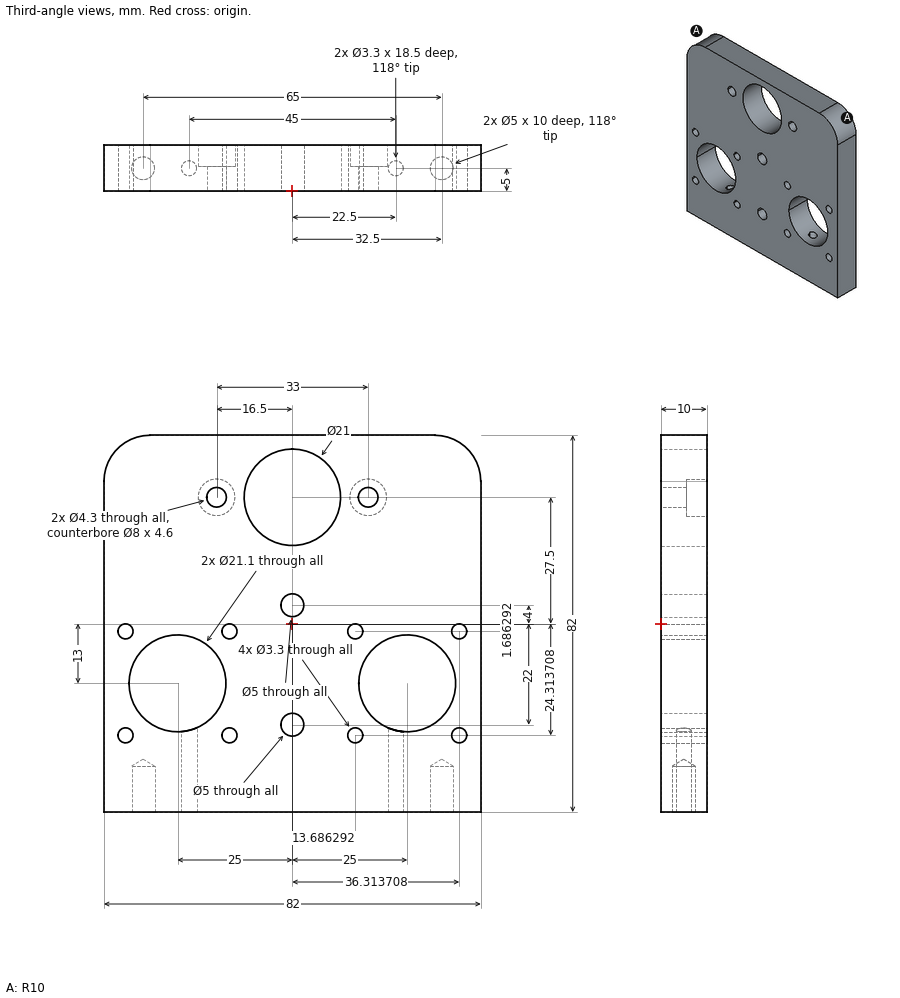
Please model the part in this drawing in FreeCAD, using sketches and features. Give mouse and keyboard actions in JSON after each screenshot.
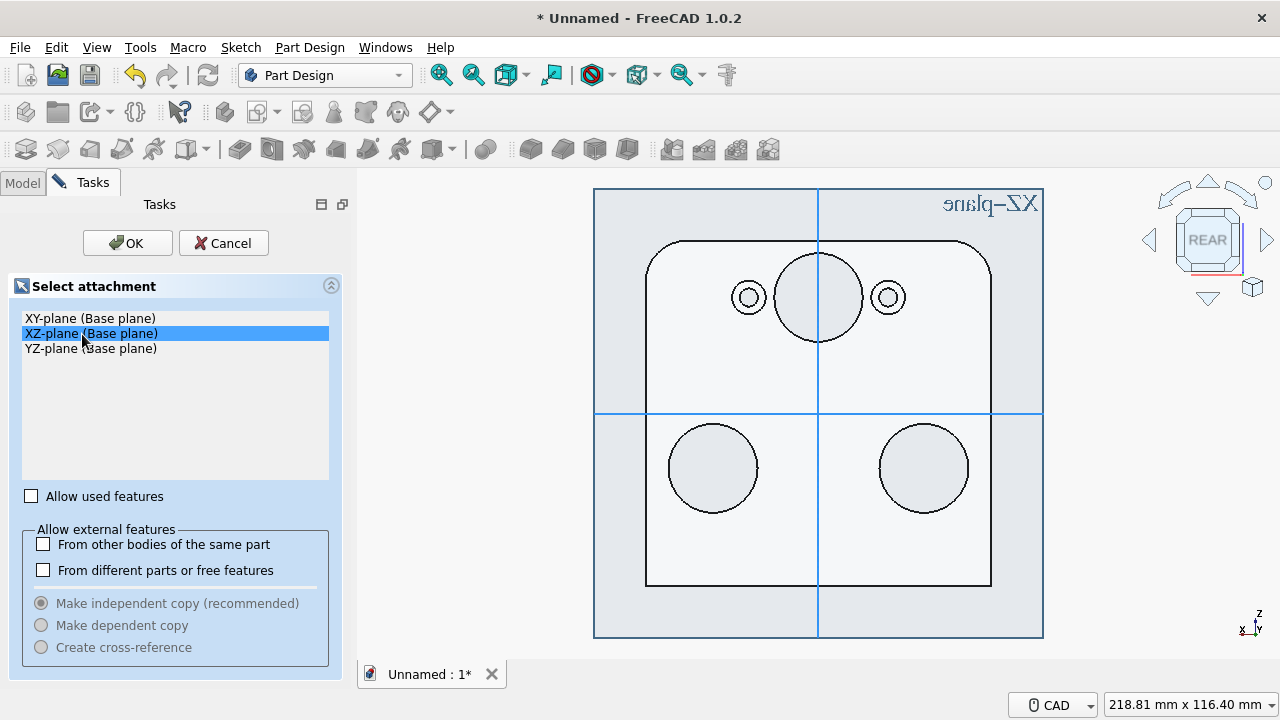
{"action": "left_click", "coordinate": [128, 243]}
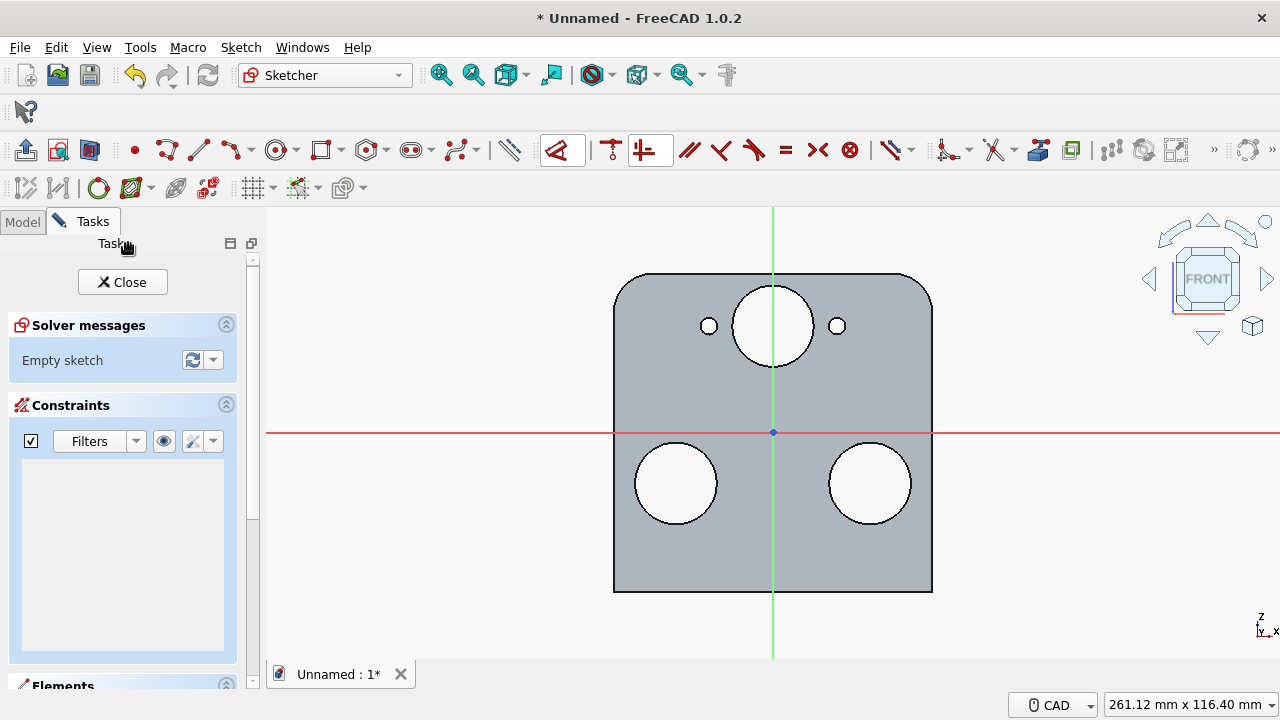
{"action": "scroll", "coordinate": [929, 513], "scroll_direction": "up", "scroll_amount": 5}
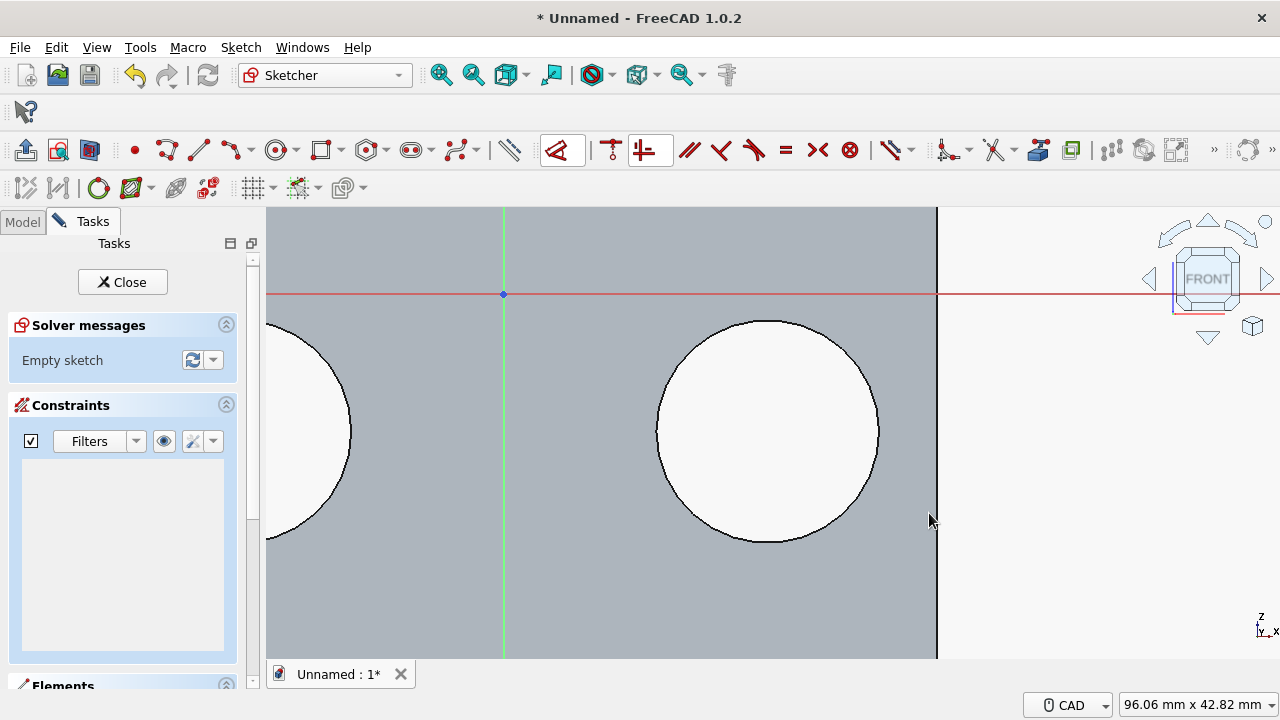
{"action": "left_click", "coordinate": [276, 150]}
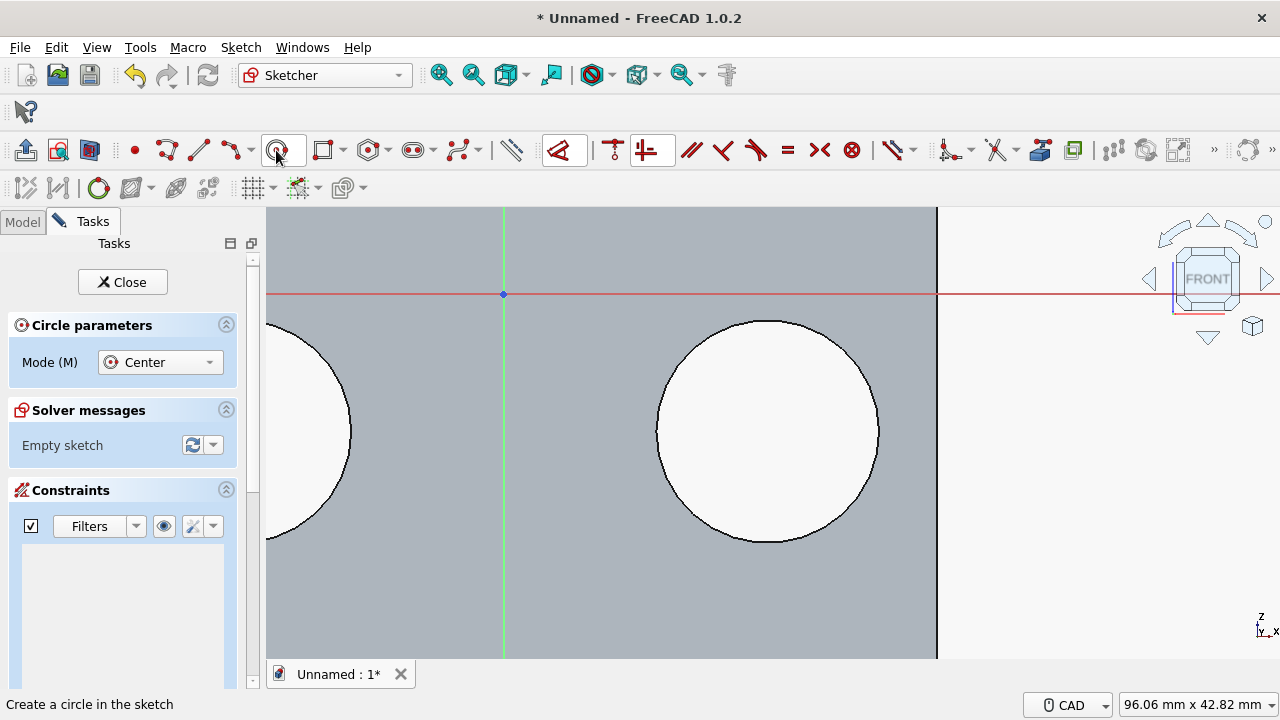
{"action": "scroll", "coordinate": [648, 551], "scroll_direction": "up", "scroll_amount": 2}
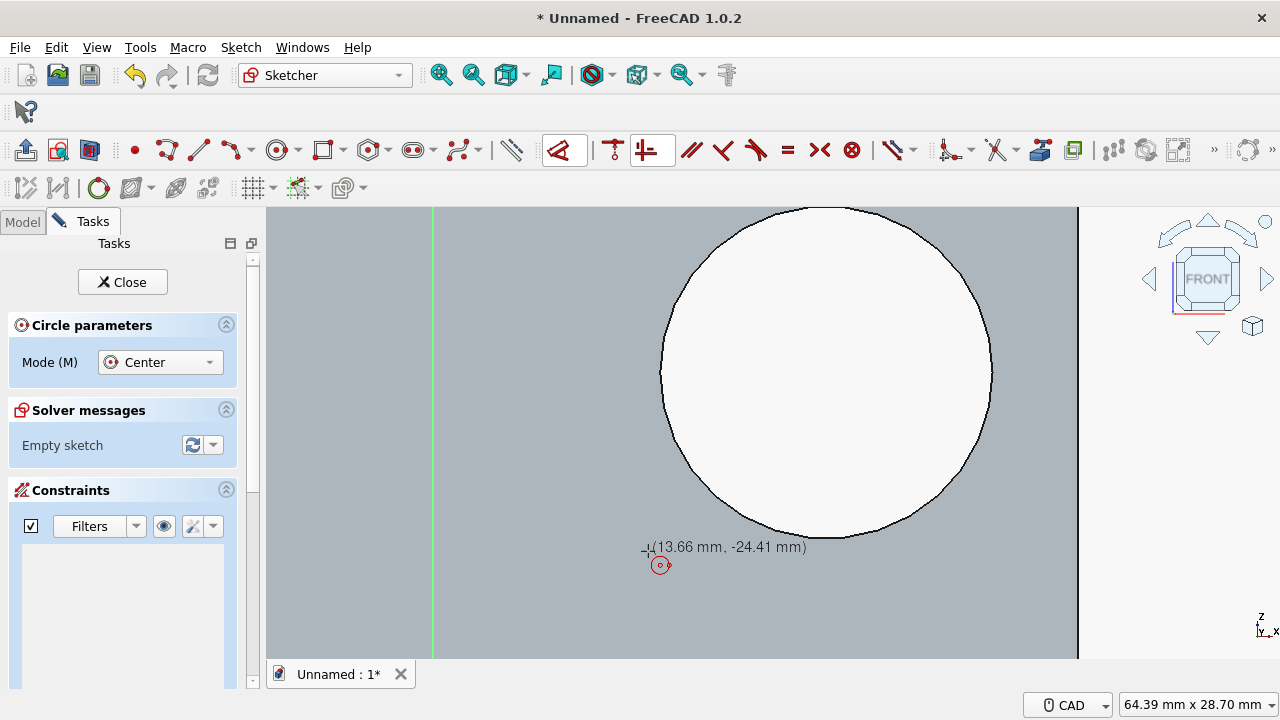
{"action": "left_click", "coordinate": [648, 551]}
{"action": "left_click", "coordinate": [667, 532]}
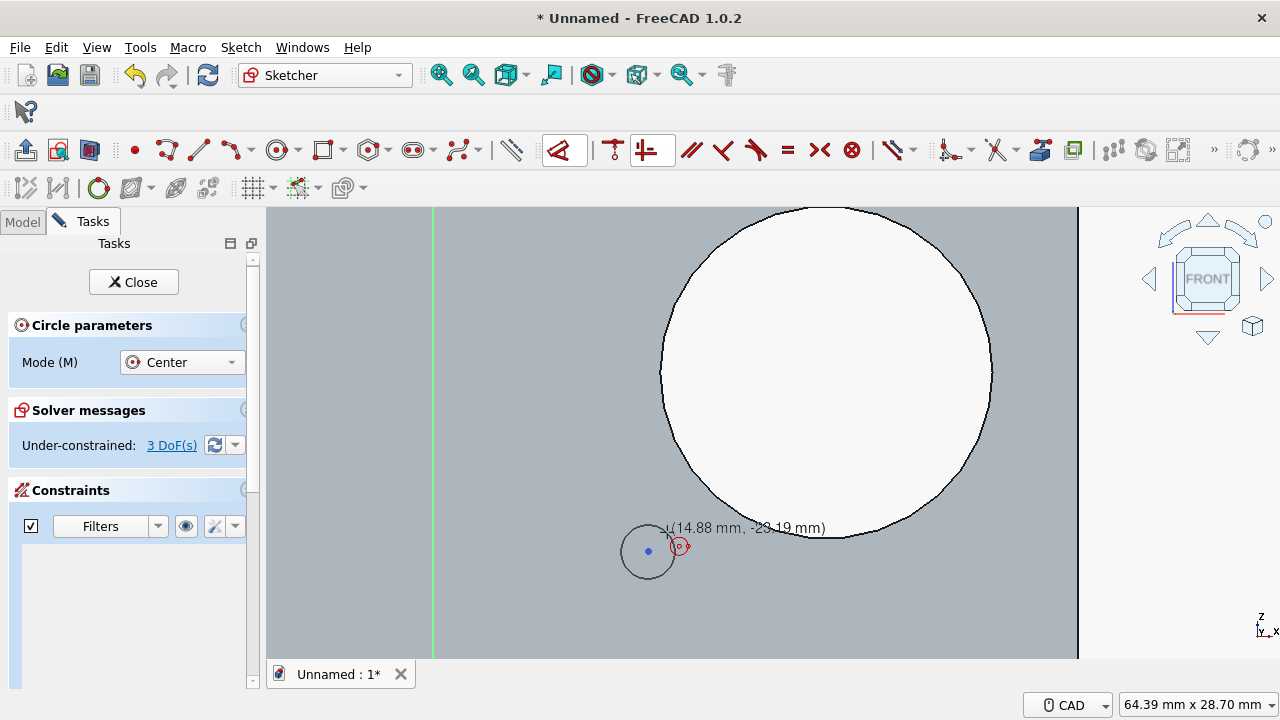
{"action": "scroll", "coordinate": [649, 557], "scroll_direction": "down", "scroll_amount": 2}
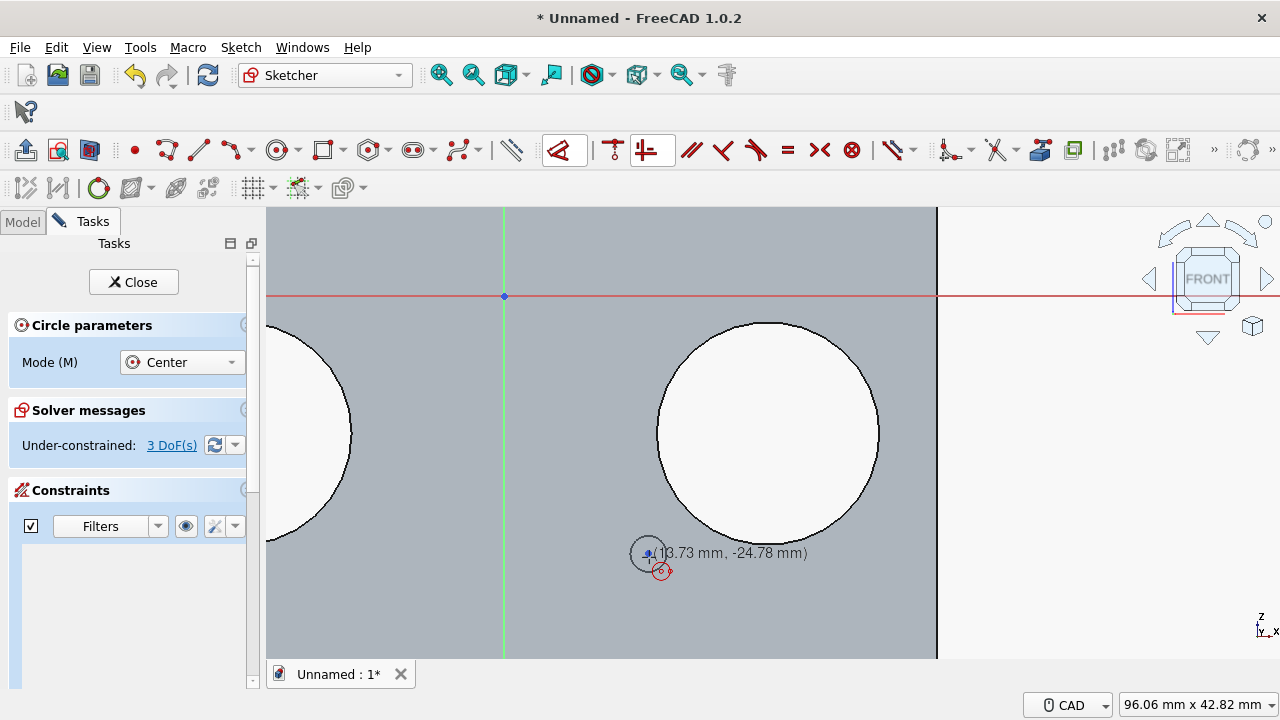
{"action": "scroll", "coordinate": [649, 314], "scroll_direction": "up", "scroll_amount": 2}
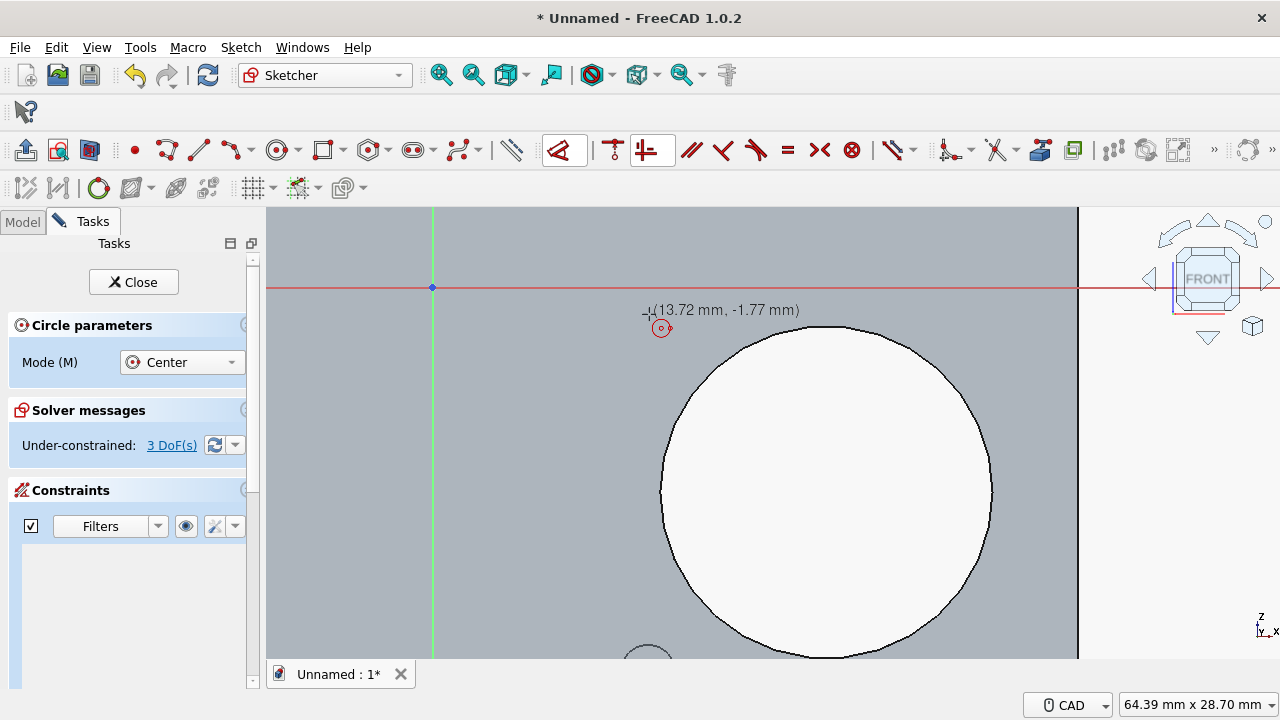
{"action": "left_click", "coordinate": [648, 314]}
{"action": "left_click", "coordinate": [667, 332]}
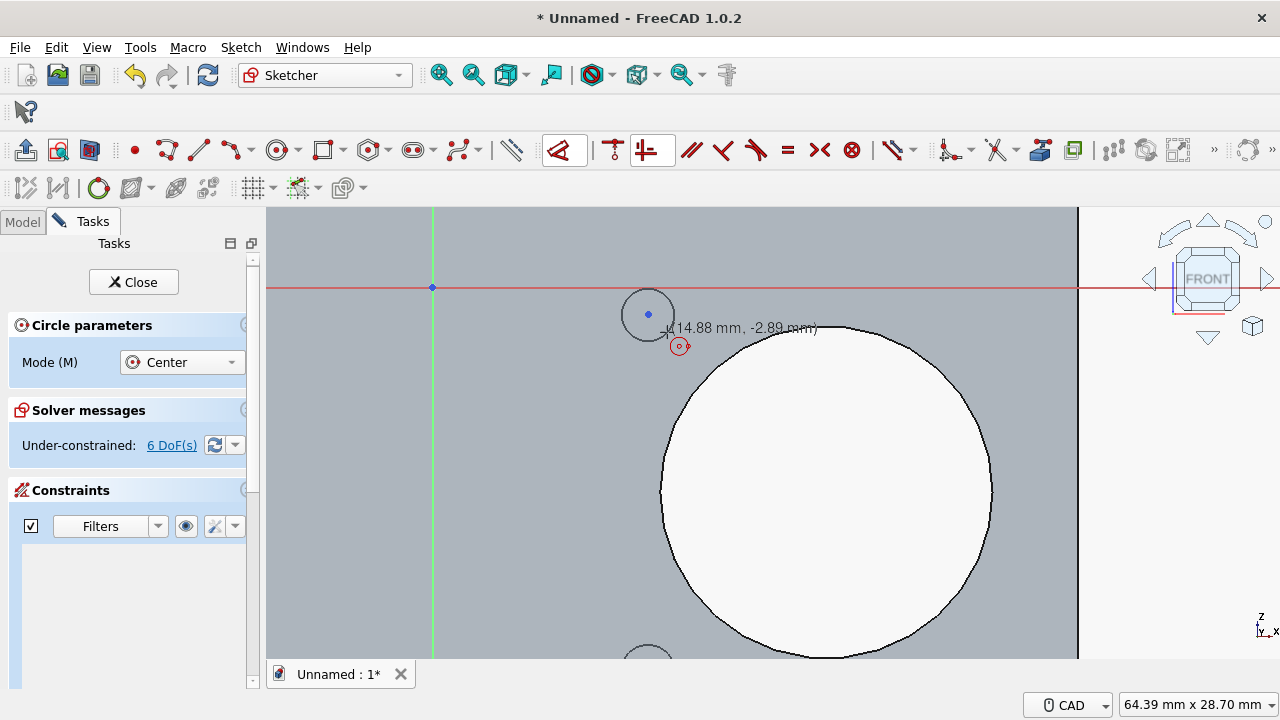
{"action": "left_click", "coordinate": [1005, 314]}
{"action": "left_click", "coordinate": [1023, 332]}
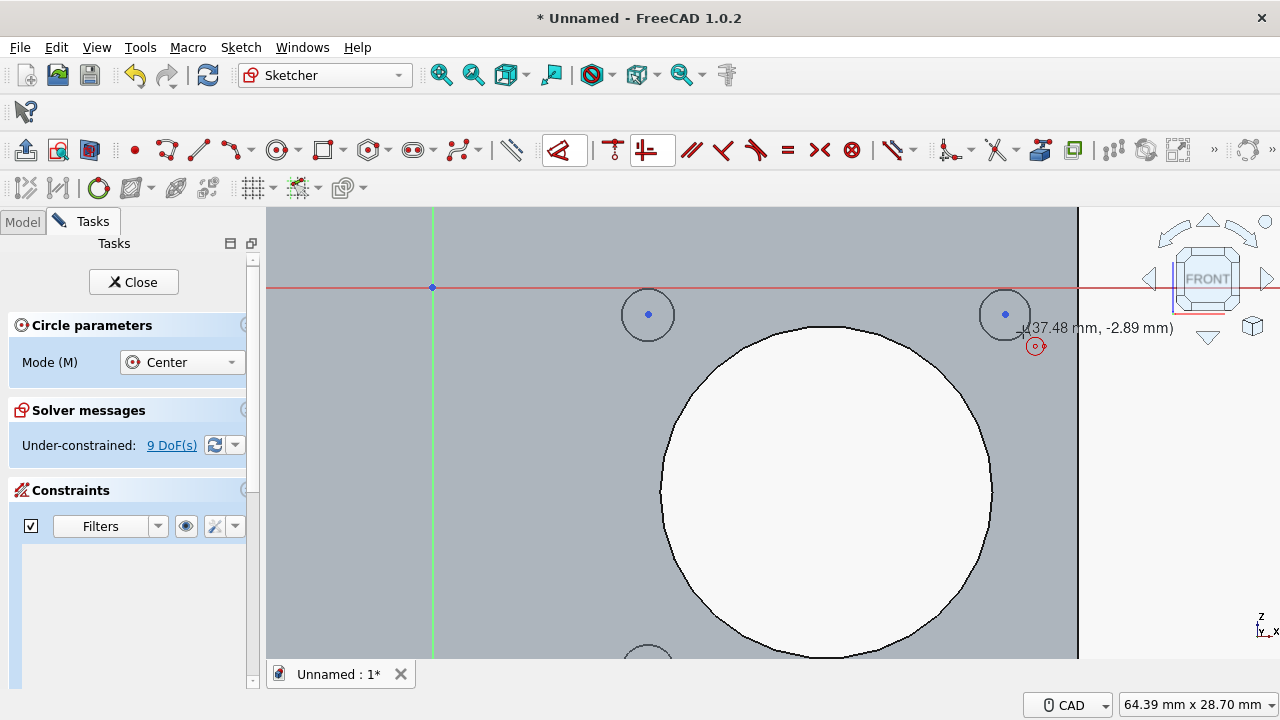
{"action": "scroll", "coordinate": [649, 313], "scroll_direction": "down", "scroll_amount": 2}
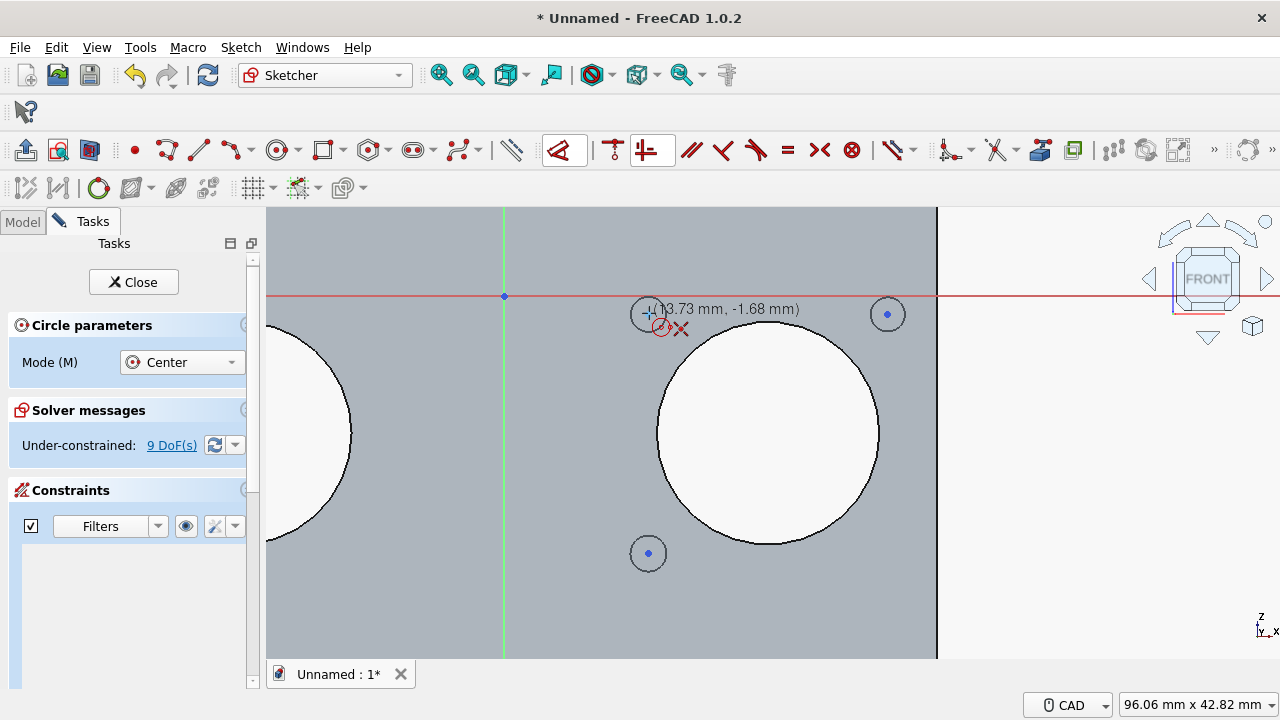
{"action": "scroll", "coordinate": [887, 553], "scroll_direction": "up", "scroll_amount": 2}